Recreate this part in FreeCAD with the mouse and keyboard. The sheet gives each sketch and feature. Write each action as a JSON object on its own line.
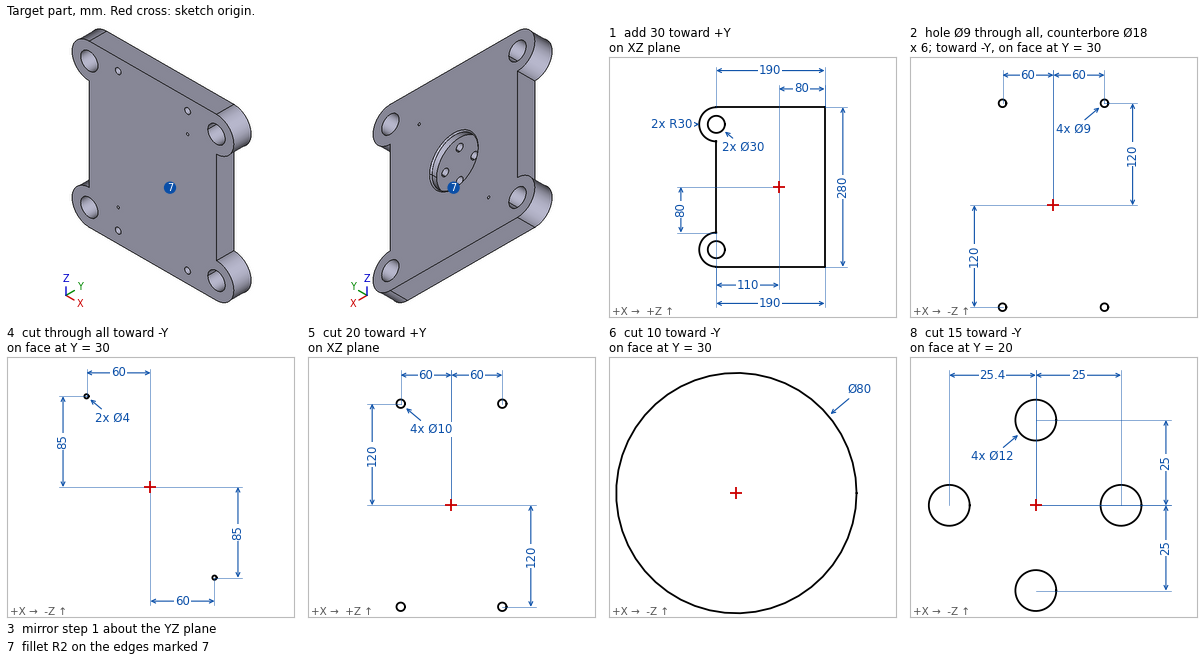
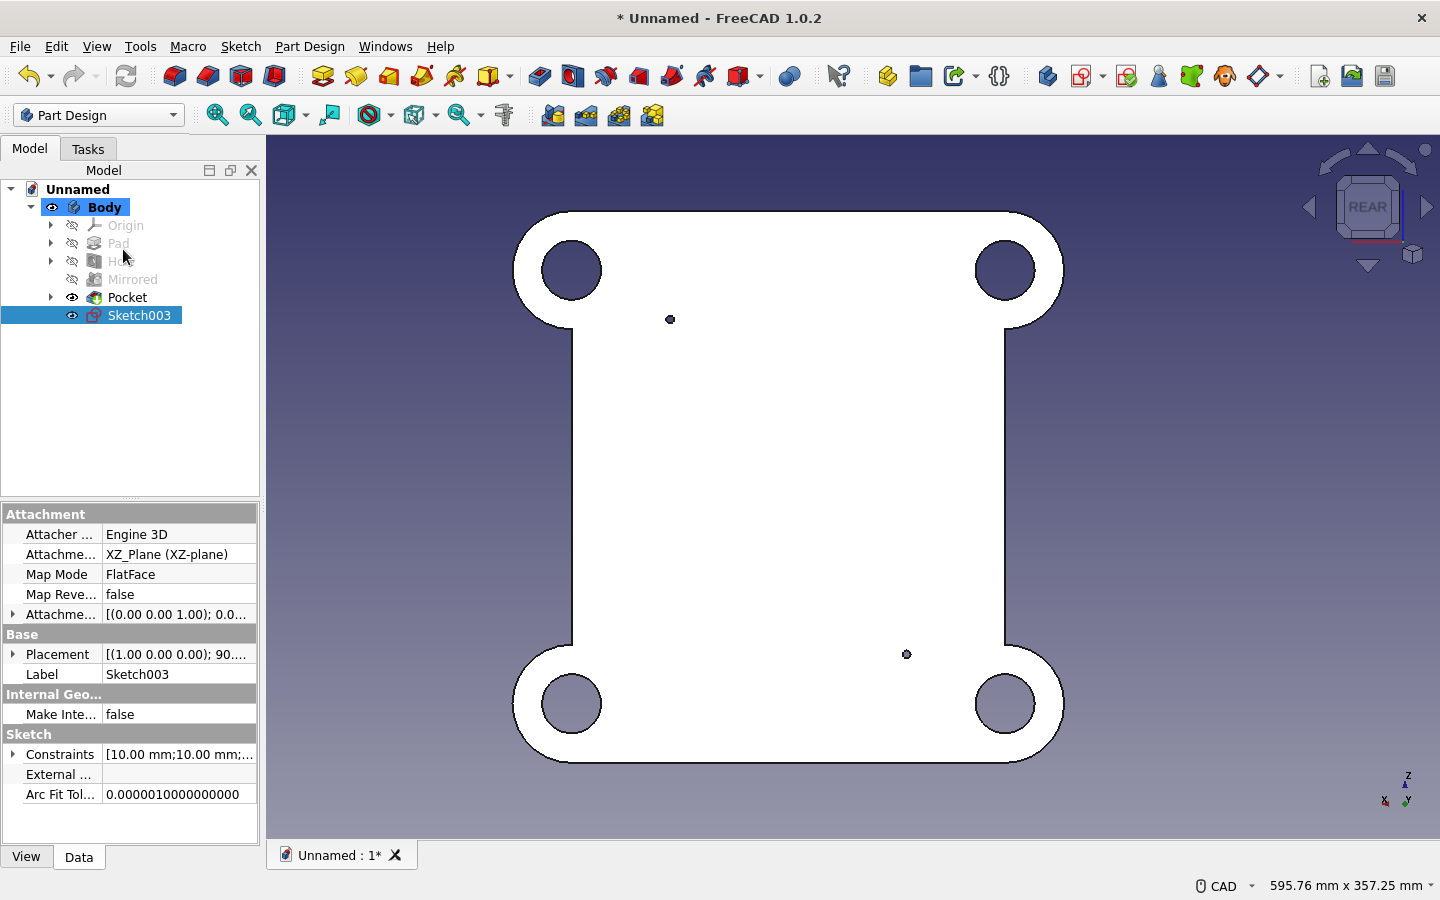
{"action": "left_click", "coordinate": [540, 76]}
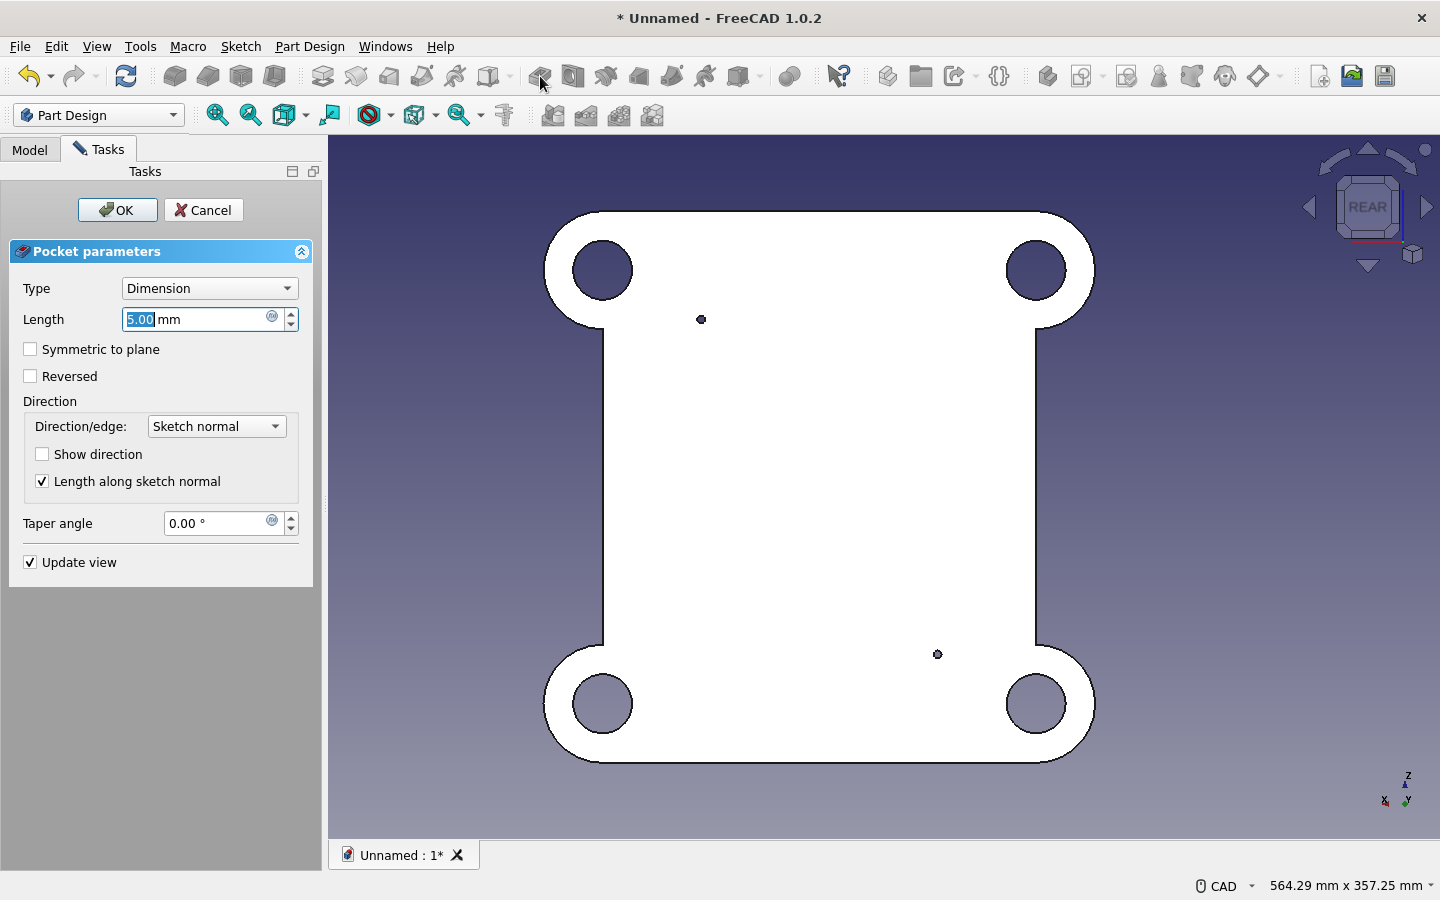
{"action": "type", "text": "20"}
{"action": "key", "text": "Tab"}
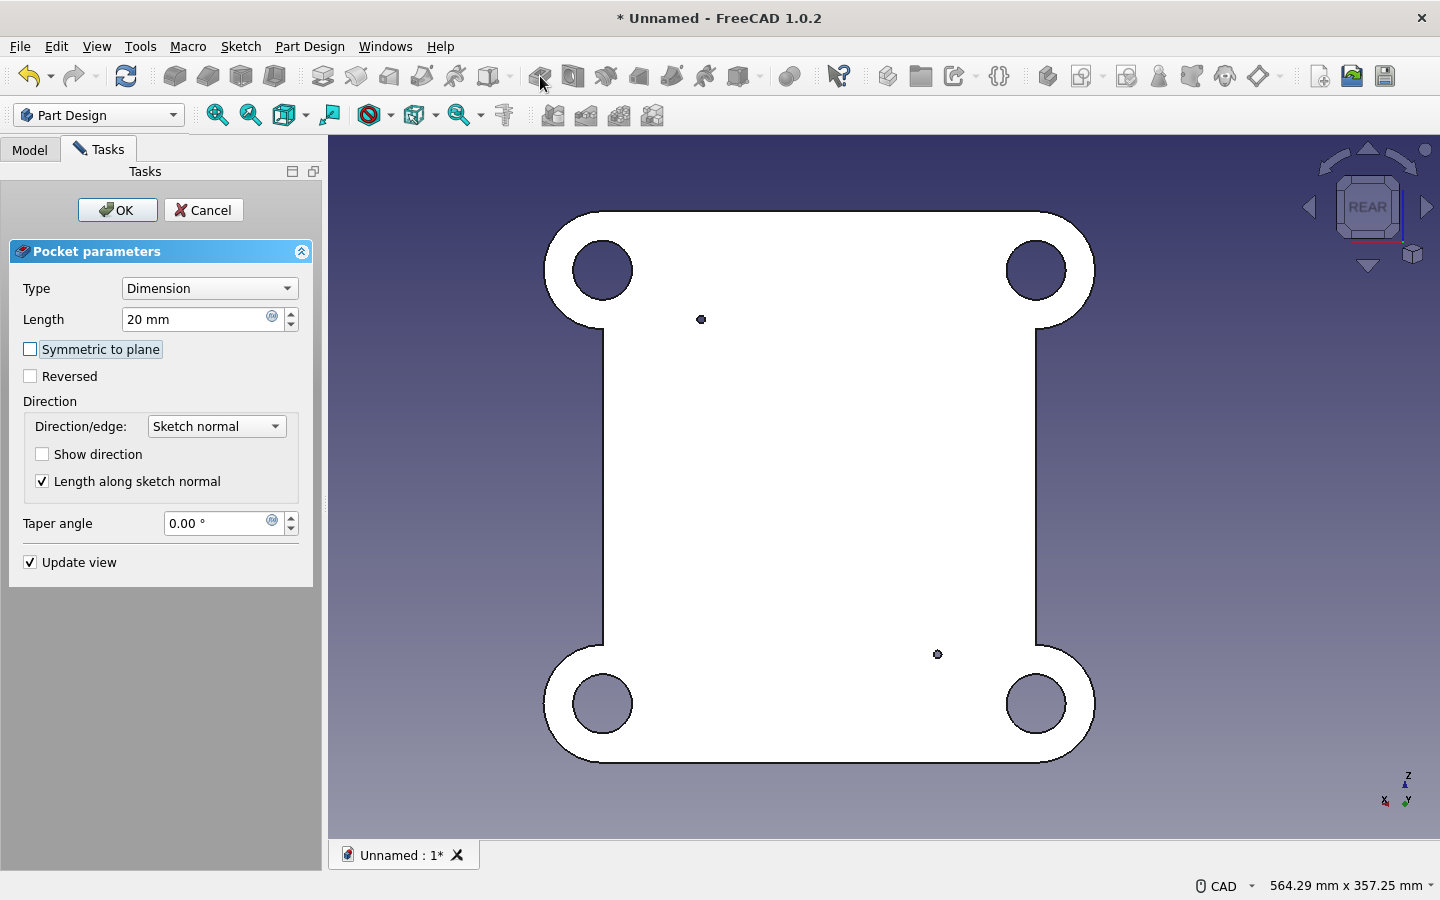
{"action": "left_click", "coordinate": [118, 210]}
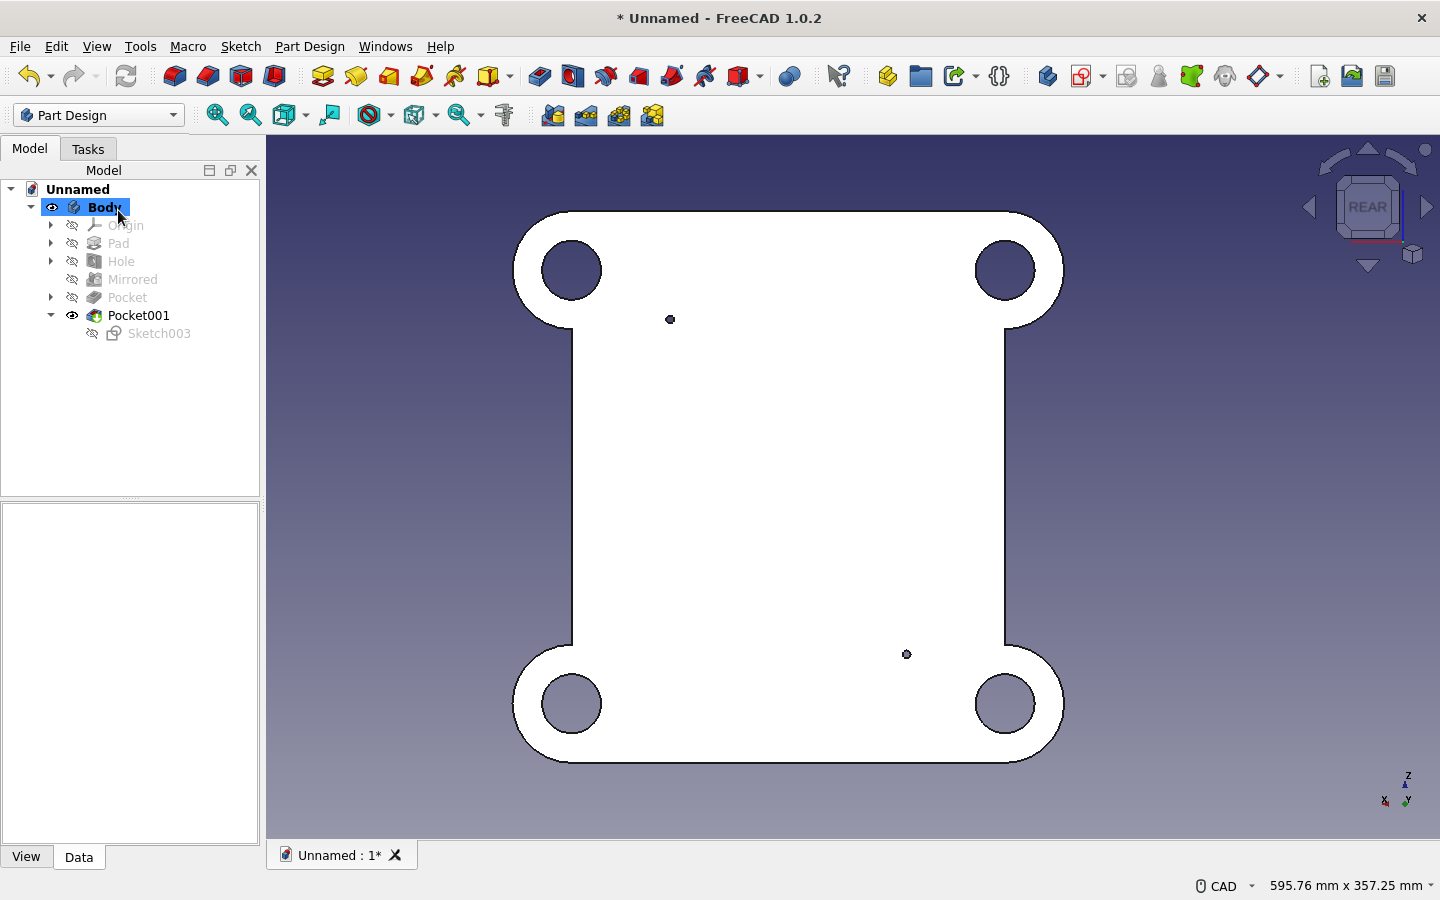
{"action": "left_click", "coordinate": [788, 486]}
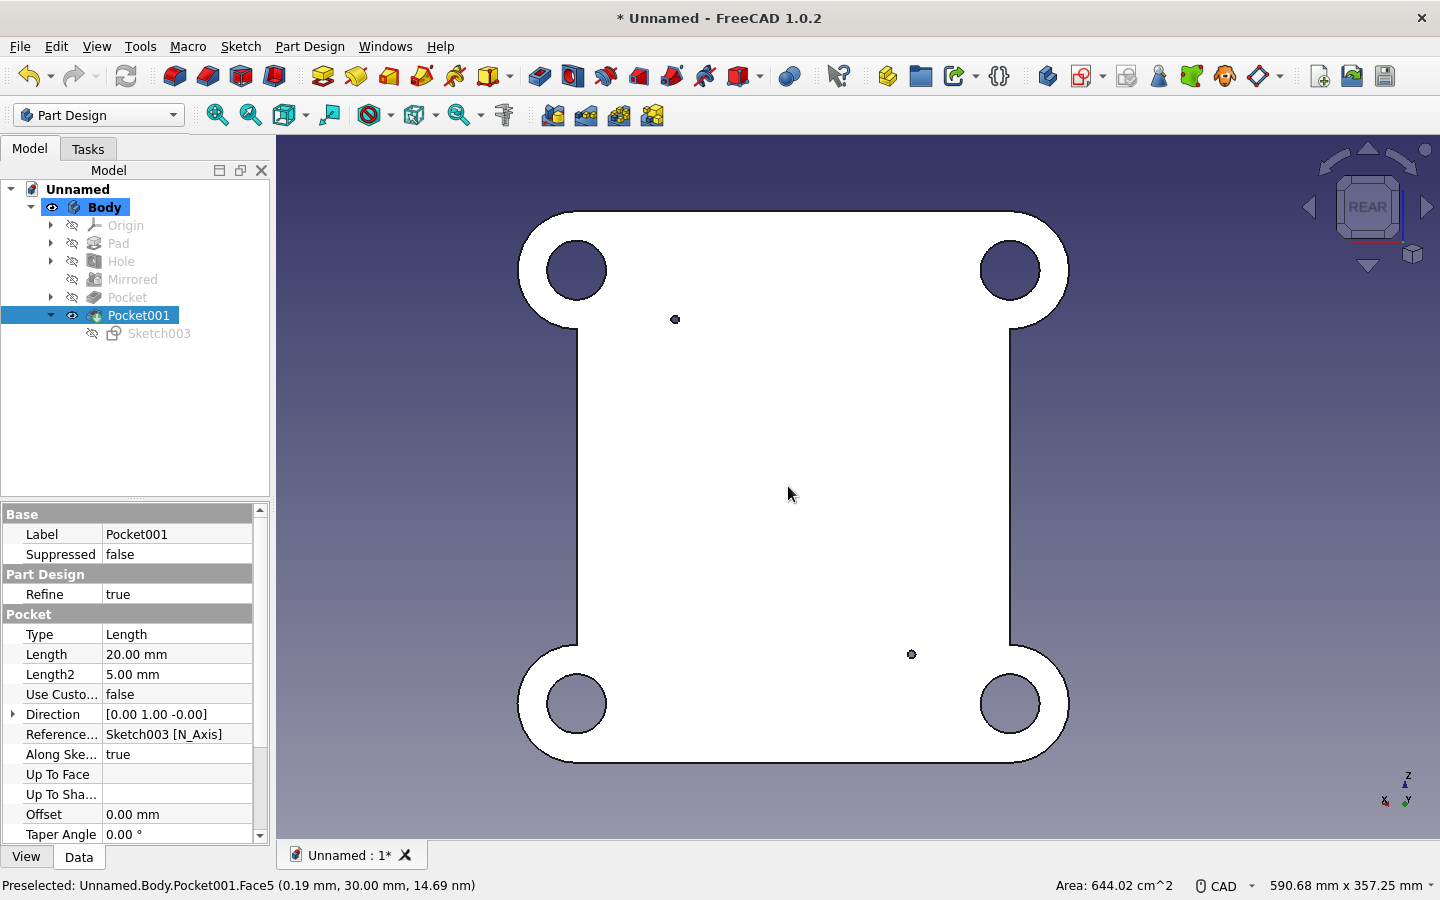
{"action": "left_click", "coordinate": [1080, 76]}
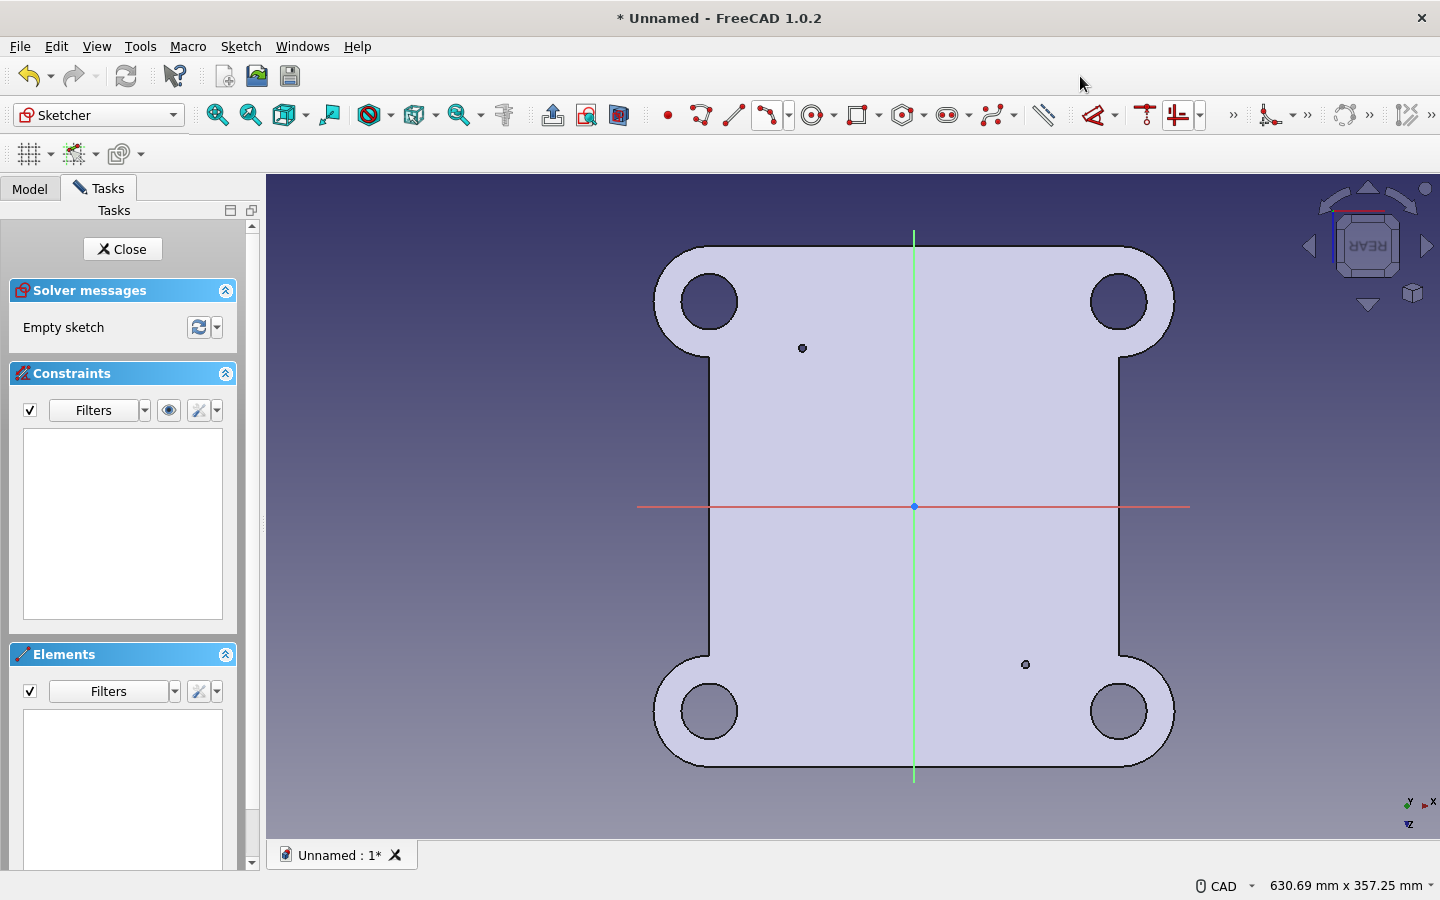
{"action": "scroll", "coordinate": [989, 506], "scroll_direction": "up", "scroll_amount": 5}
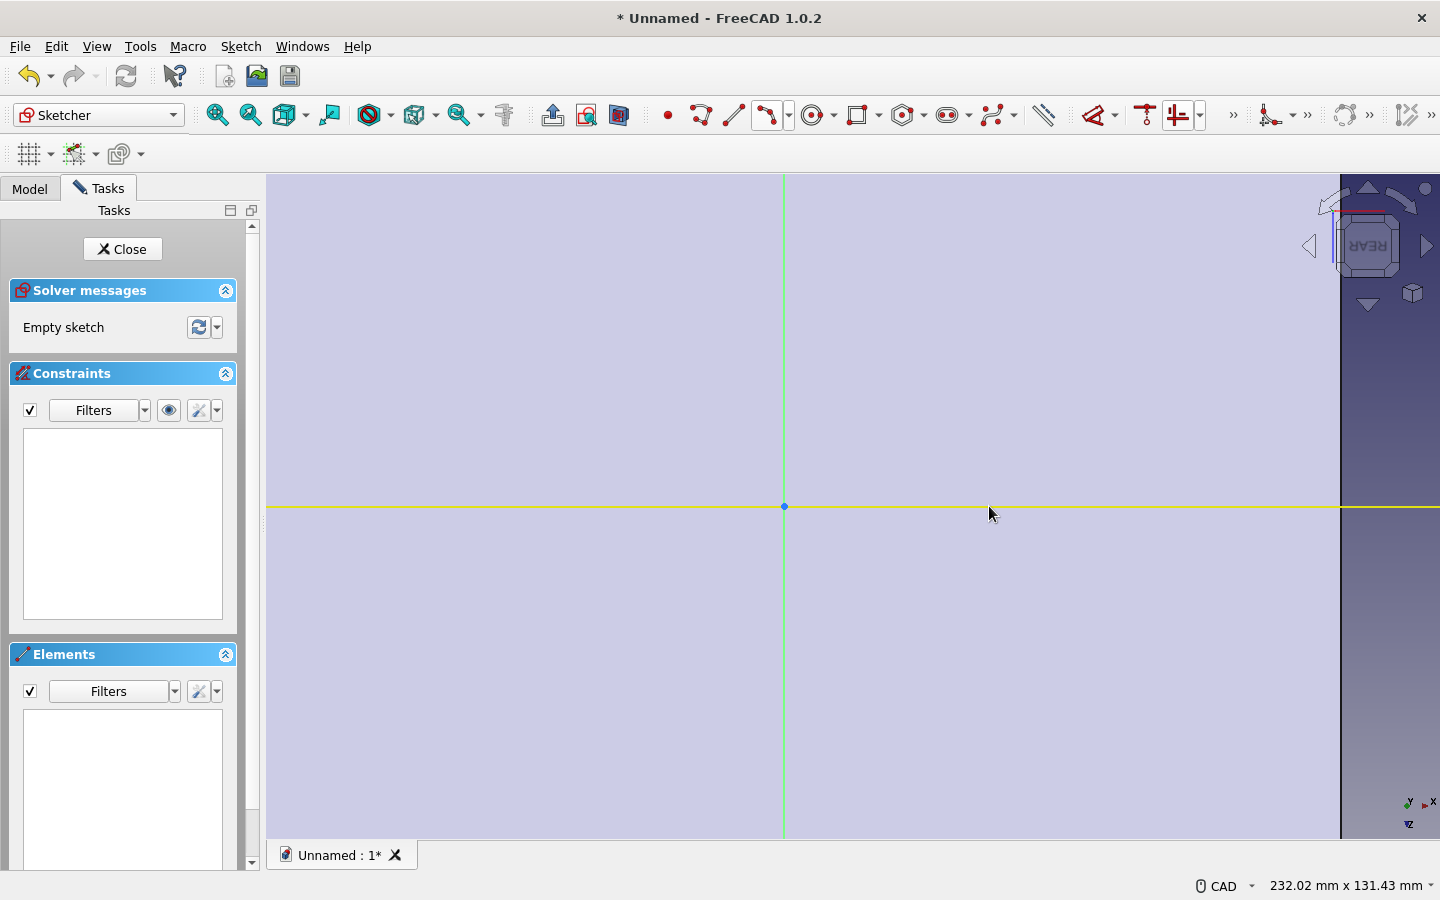
{"action": "left_click", "coordinate": [812, 116]}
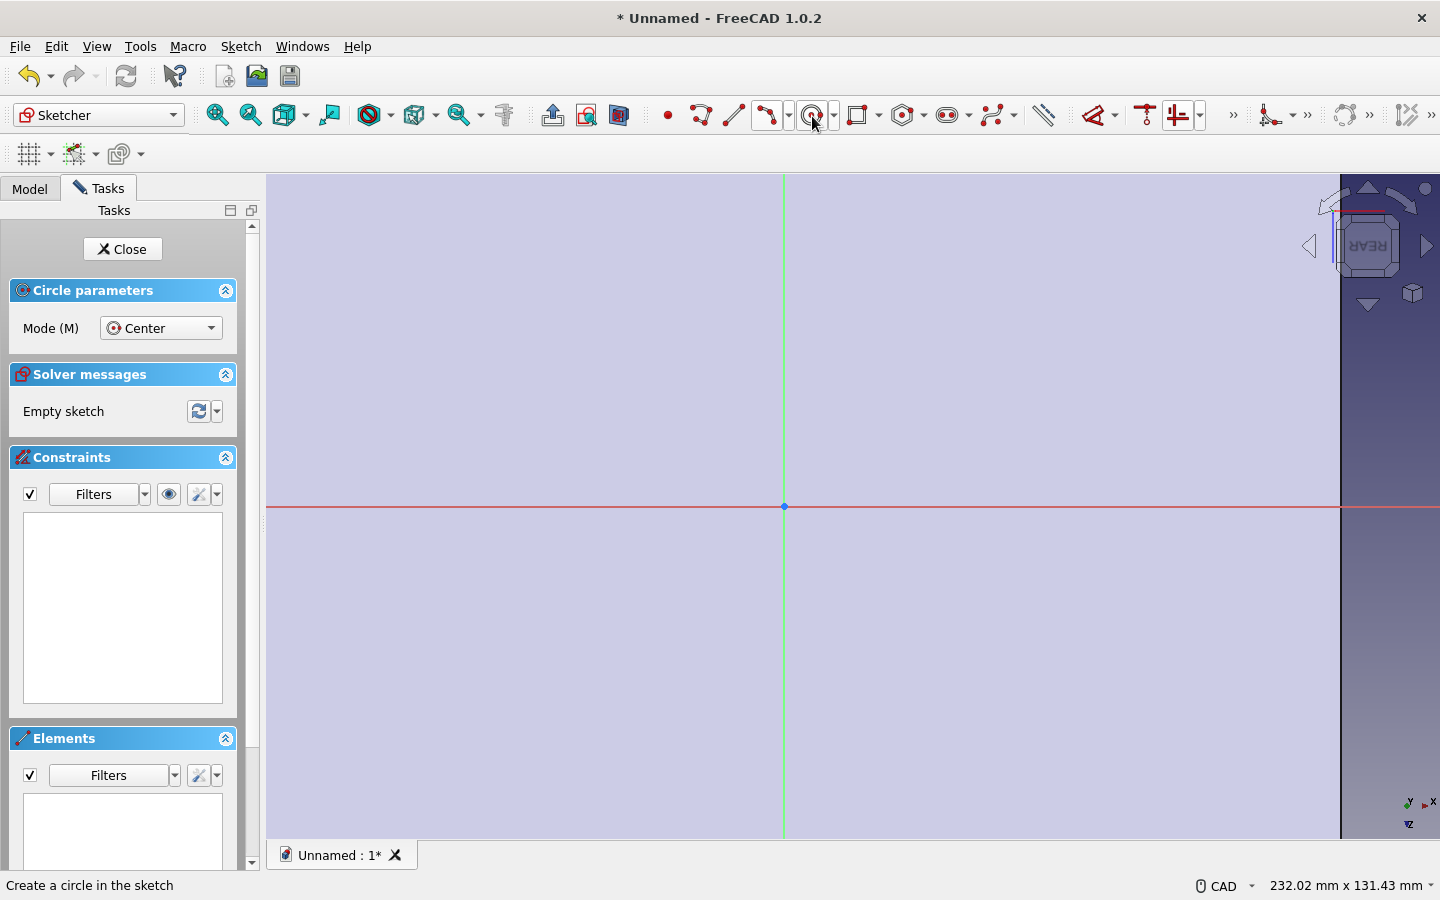
{"action": "left_click", "coordinate": [784, 506]}
{"action": "mouse_move", "coordinate": [927, 363]}